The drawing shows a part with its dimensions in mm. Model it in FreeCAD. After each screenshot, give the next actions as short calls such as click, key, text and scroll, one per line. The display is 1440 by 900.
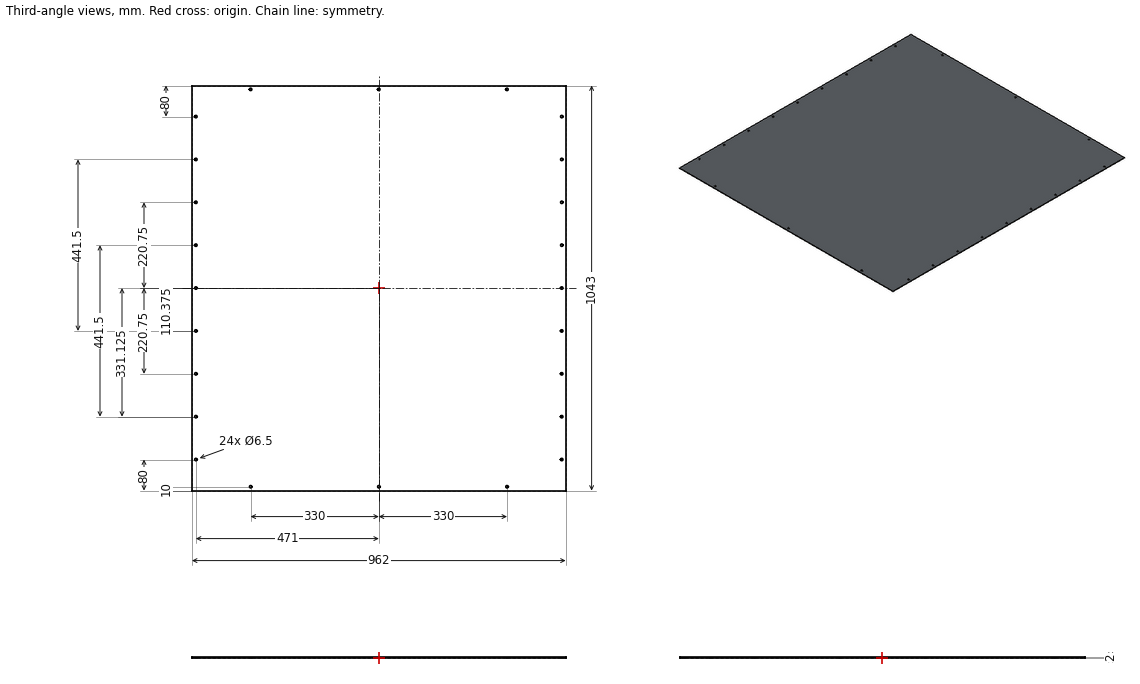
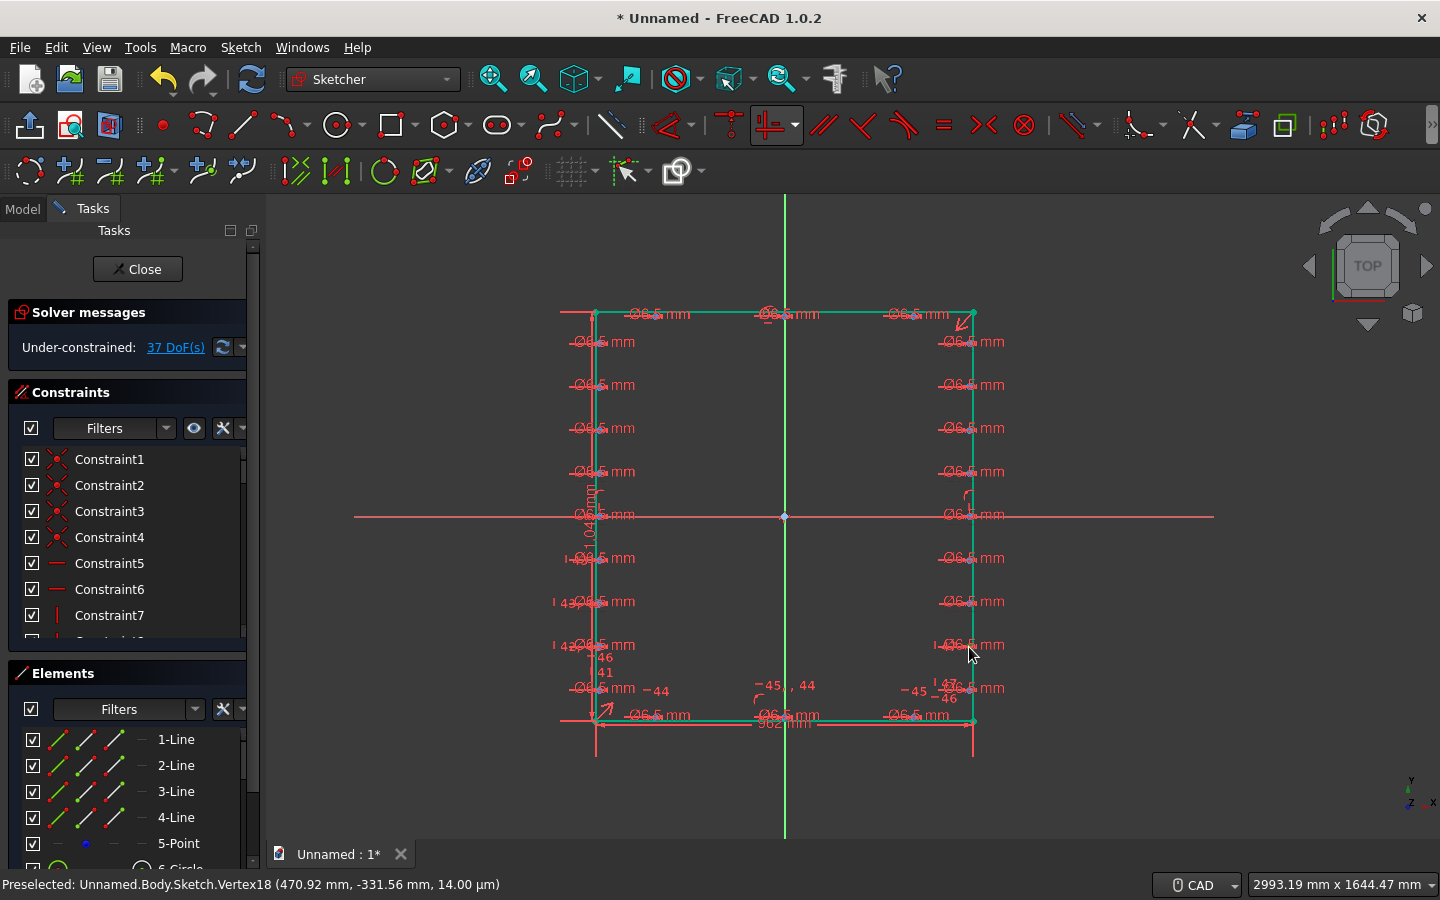
click(969, 604)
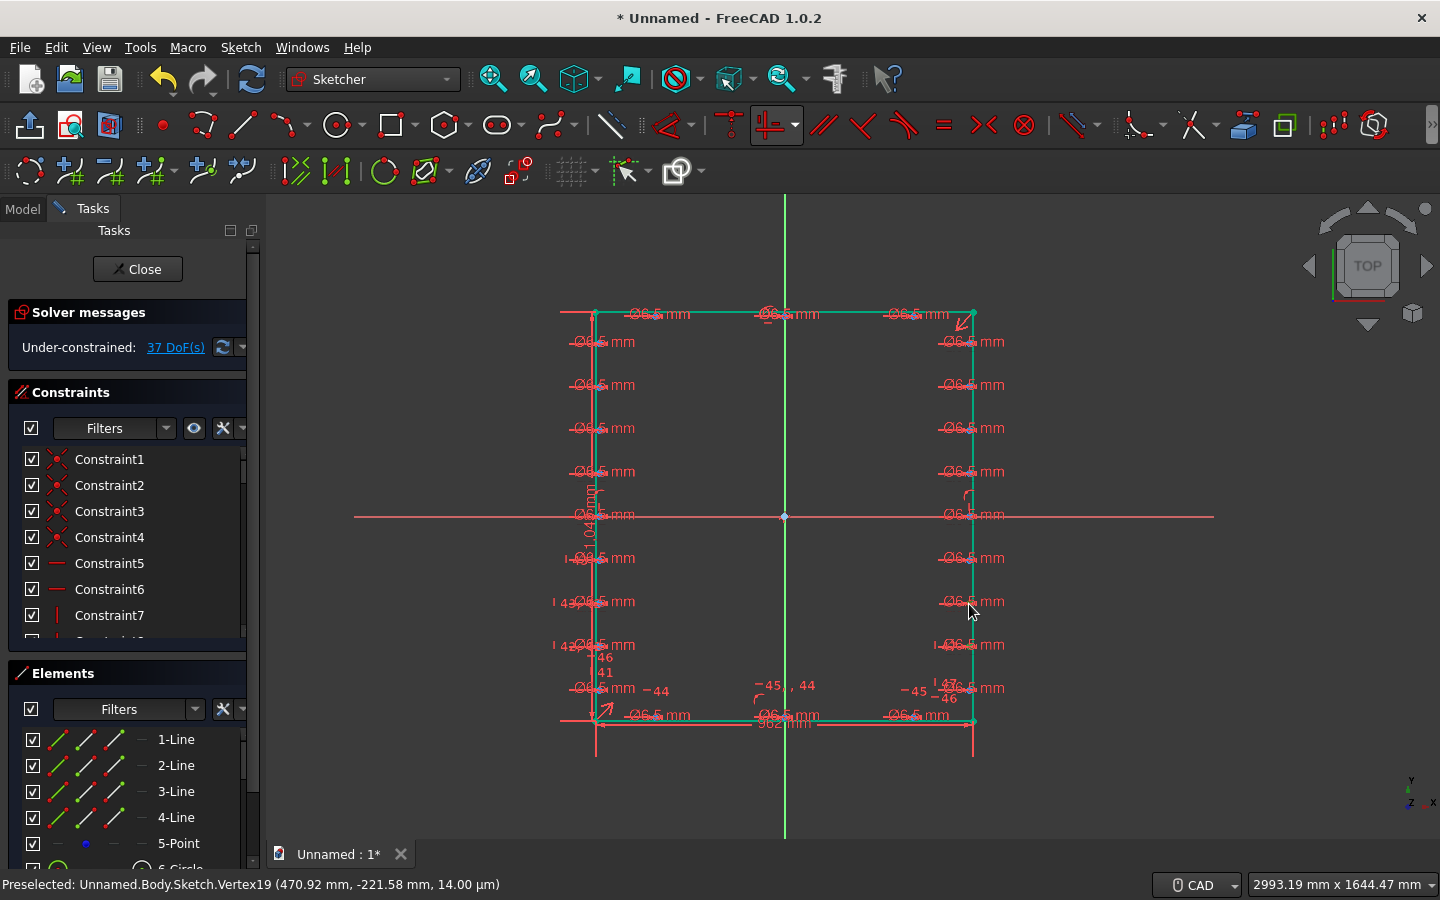
key(v)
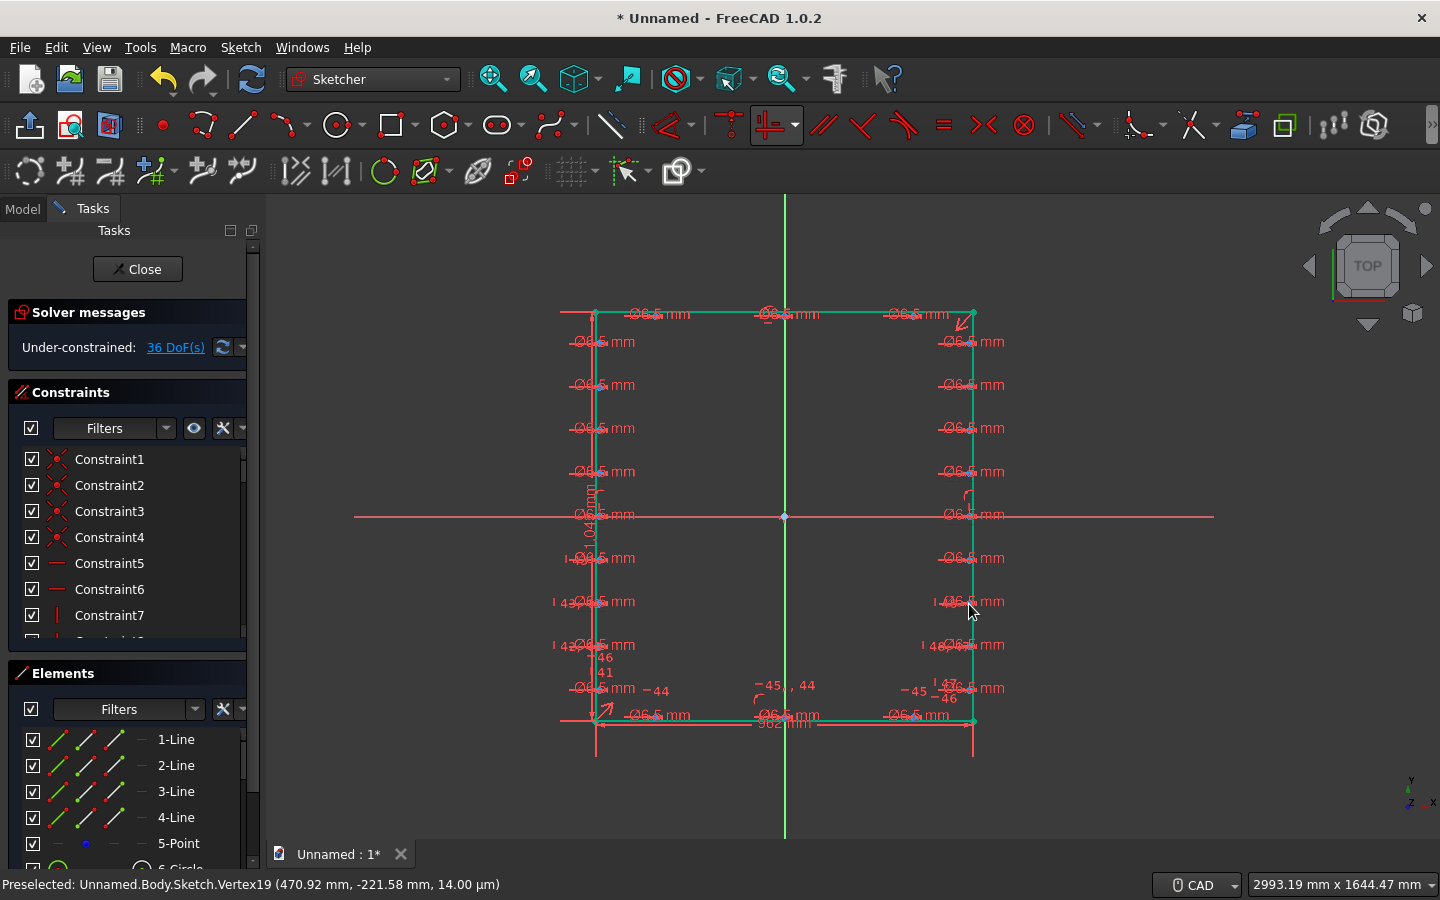
click(969, 604)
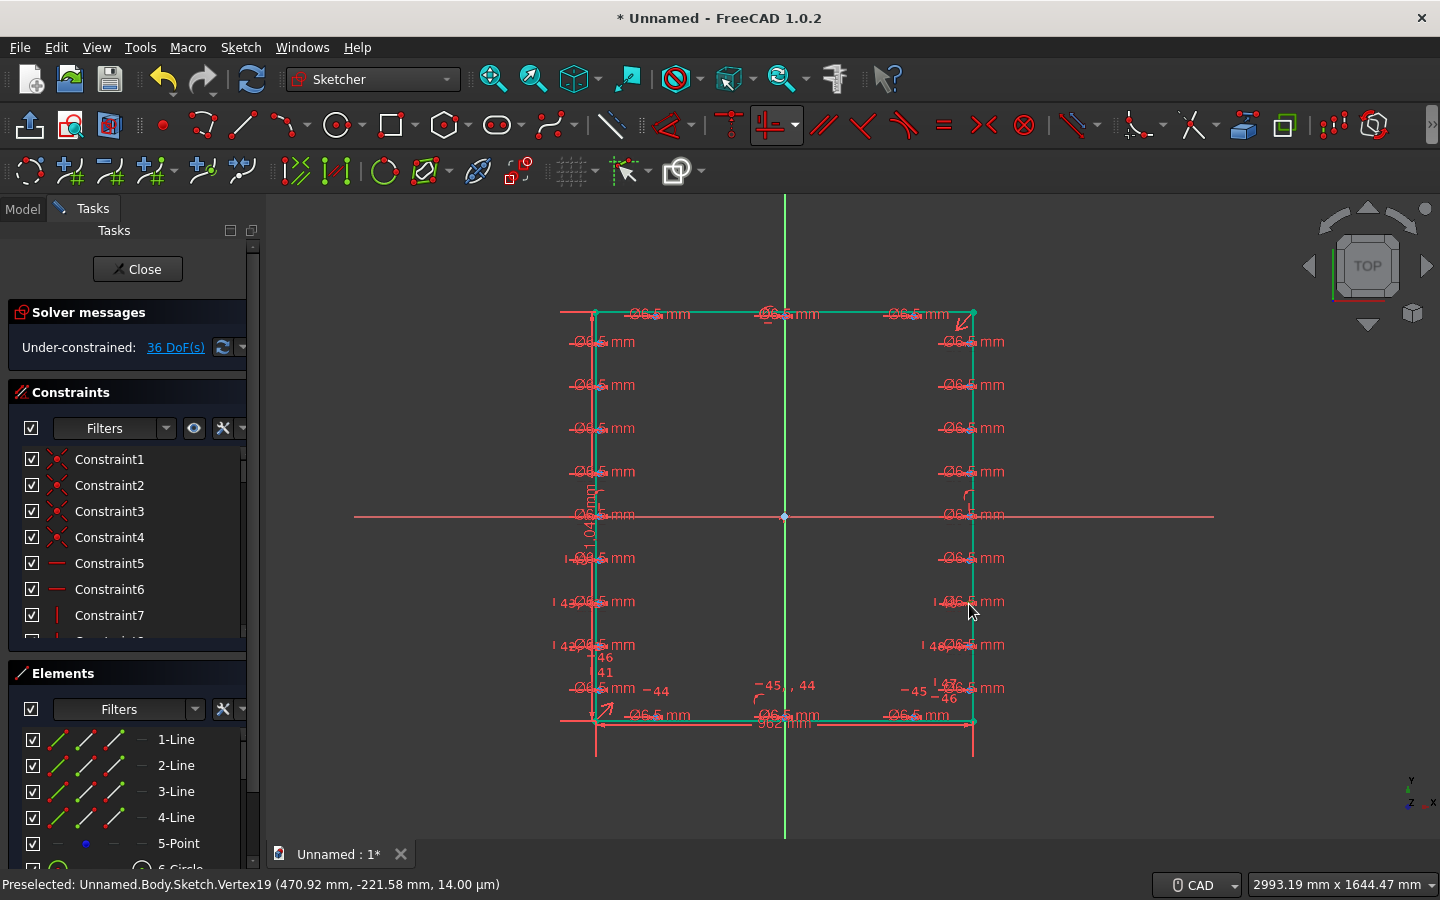
click(969, 560)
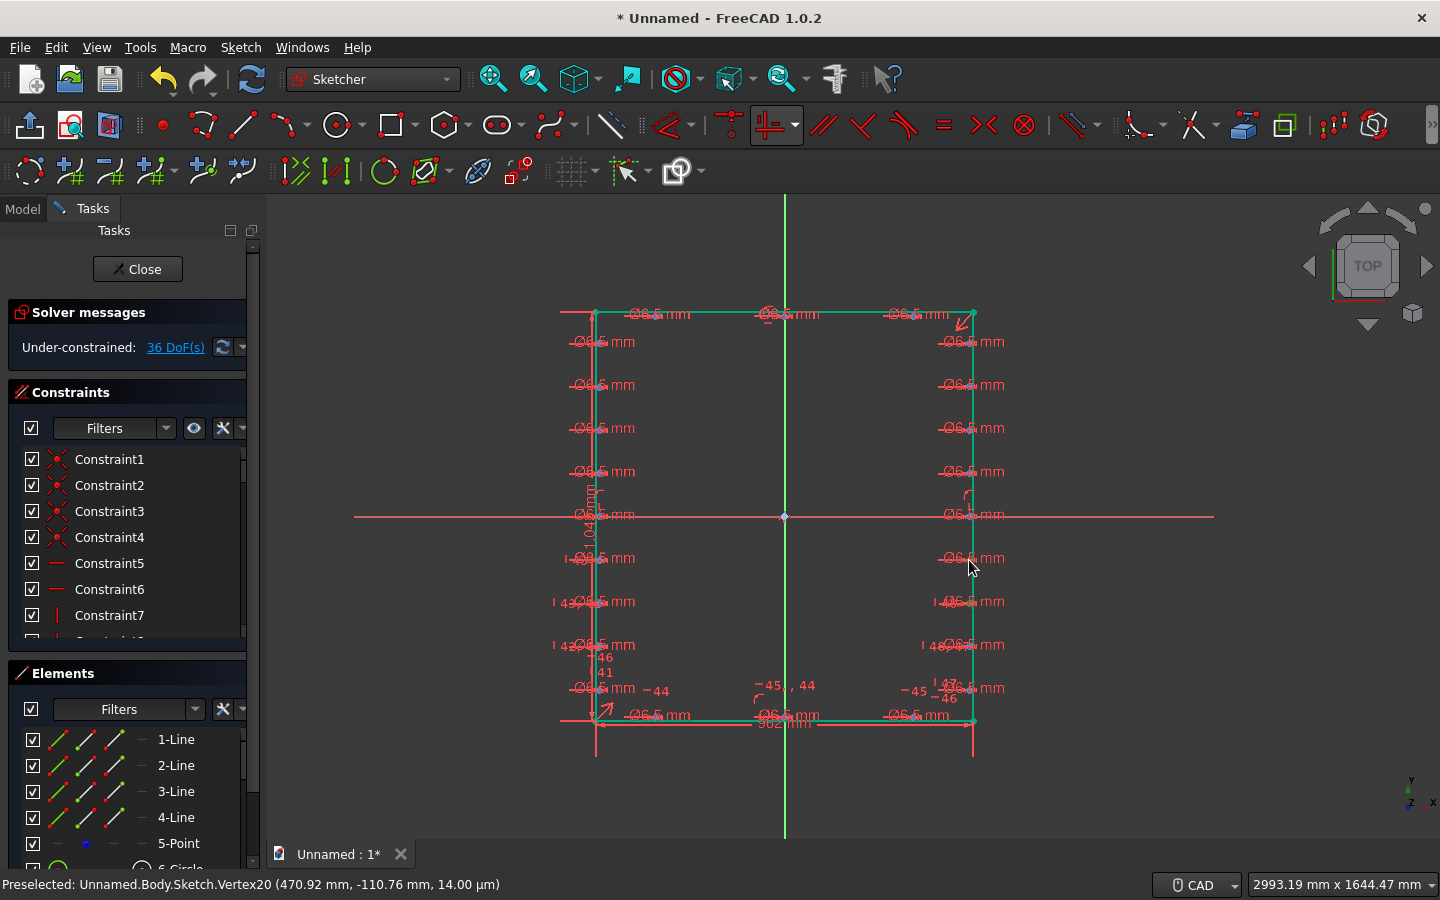
key(v)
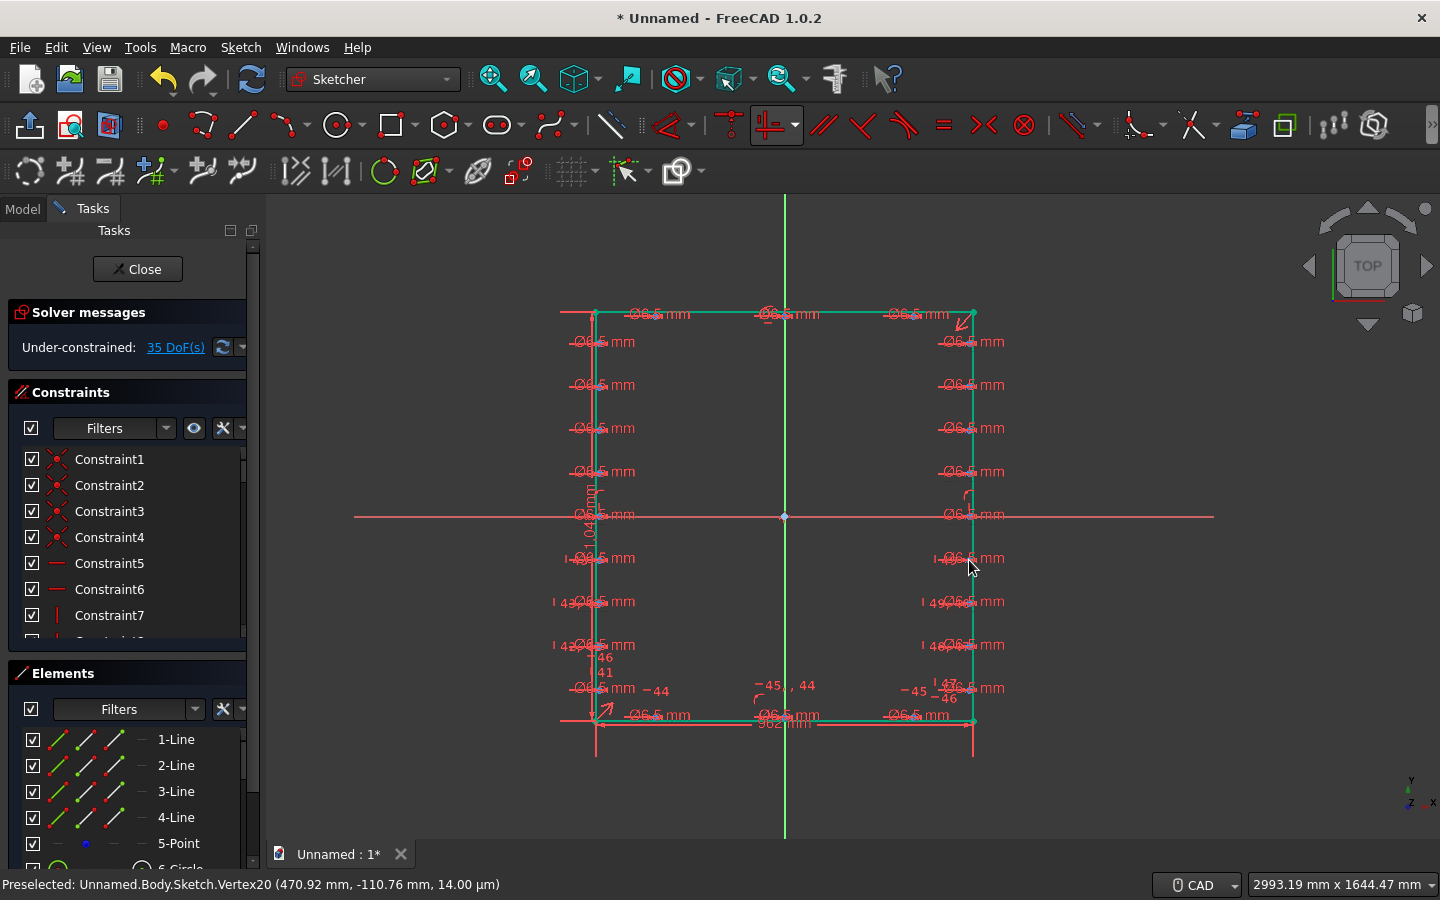
click(600, 560)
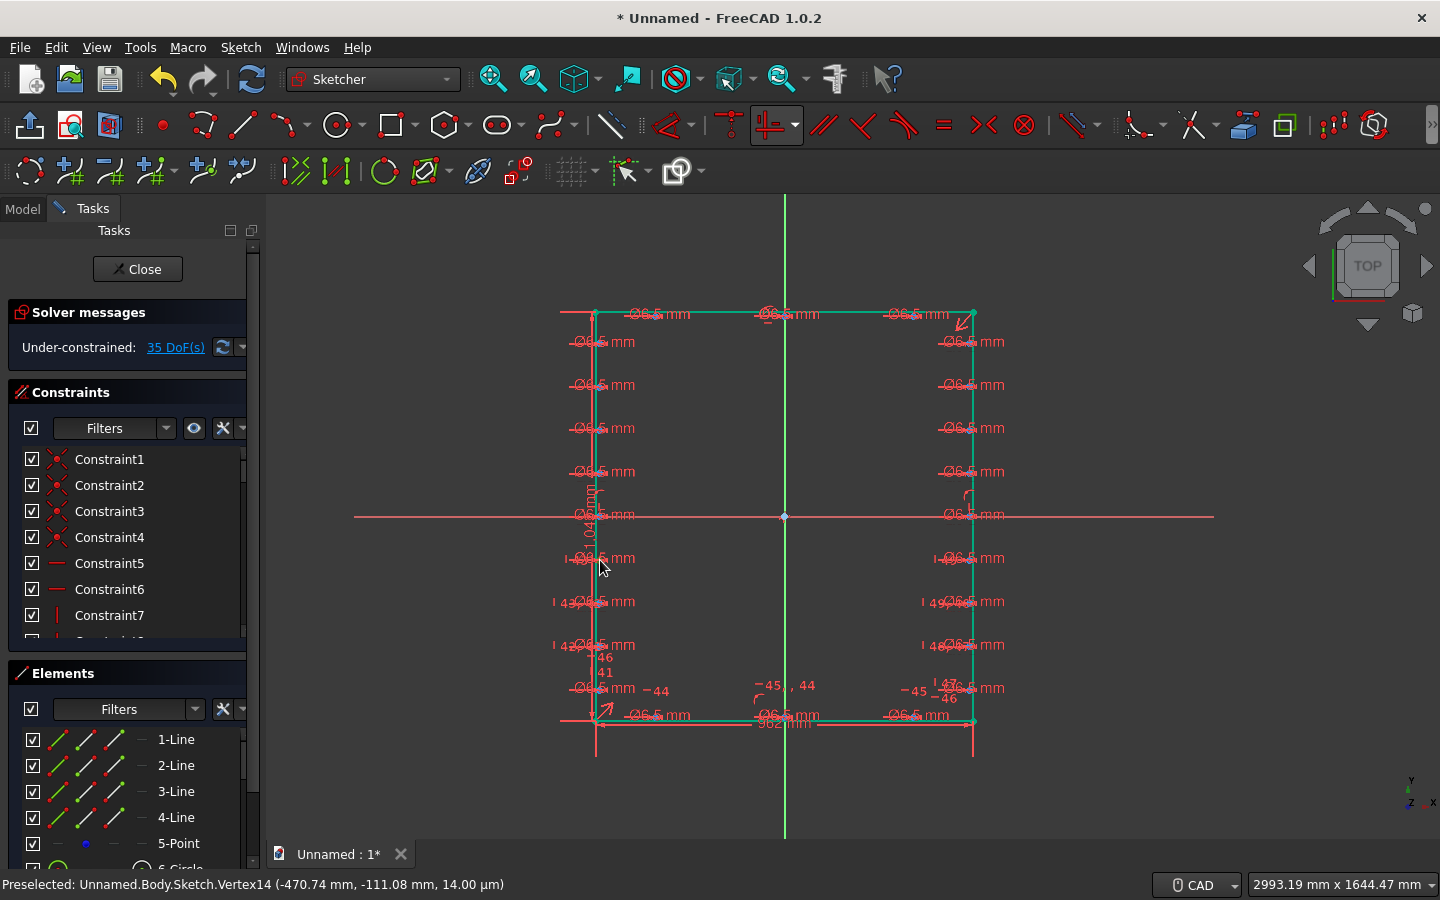
click(600, 517)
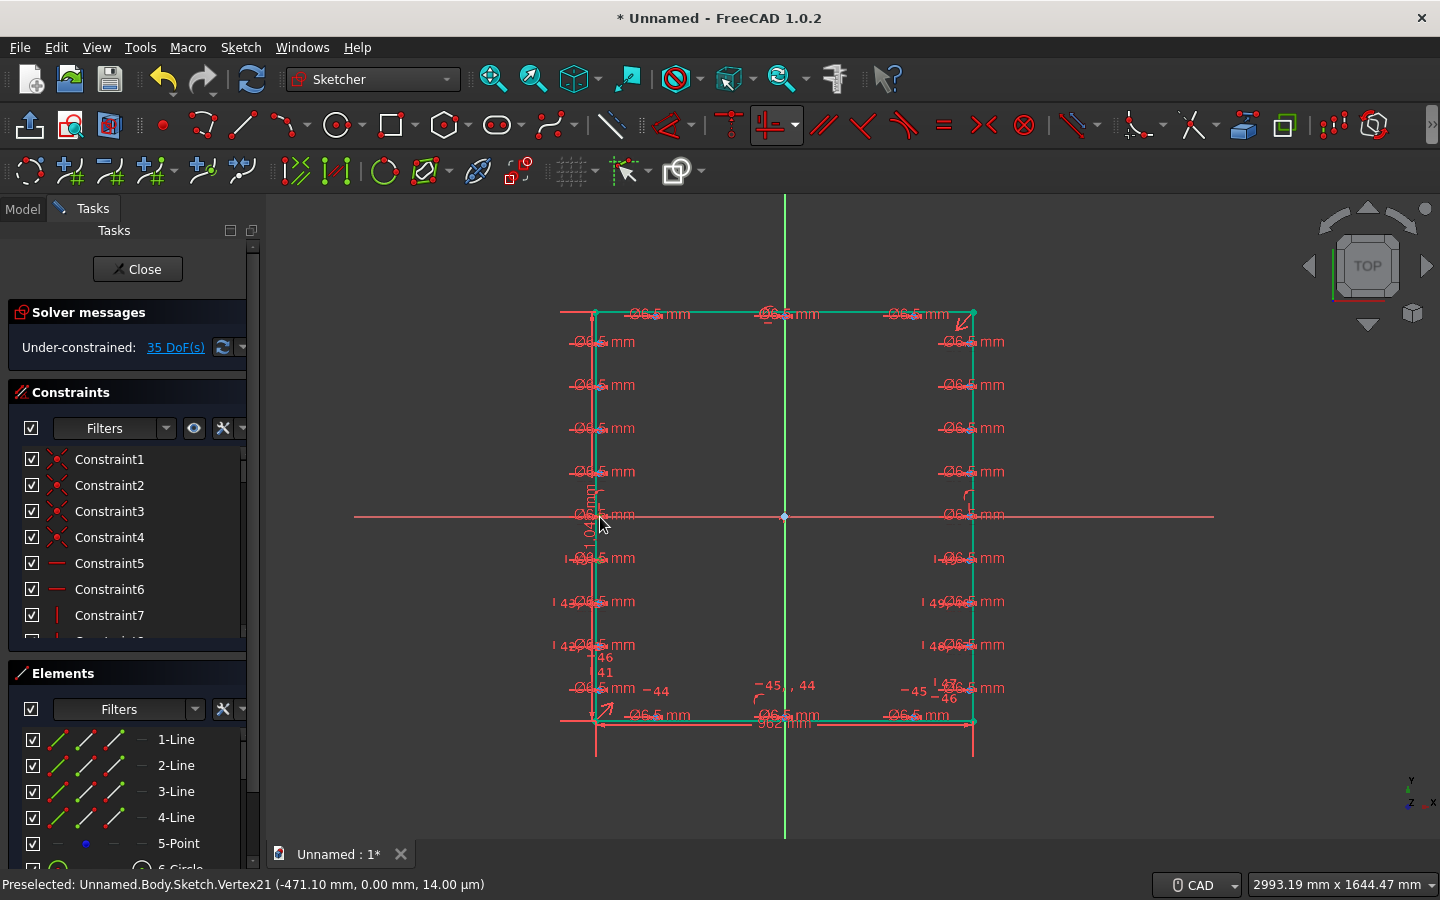
click(798, 126)